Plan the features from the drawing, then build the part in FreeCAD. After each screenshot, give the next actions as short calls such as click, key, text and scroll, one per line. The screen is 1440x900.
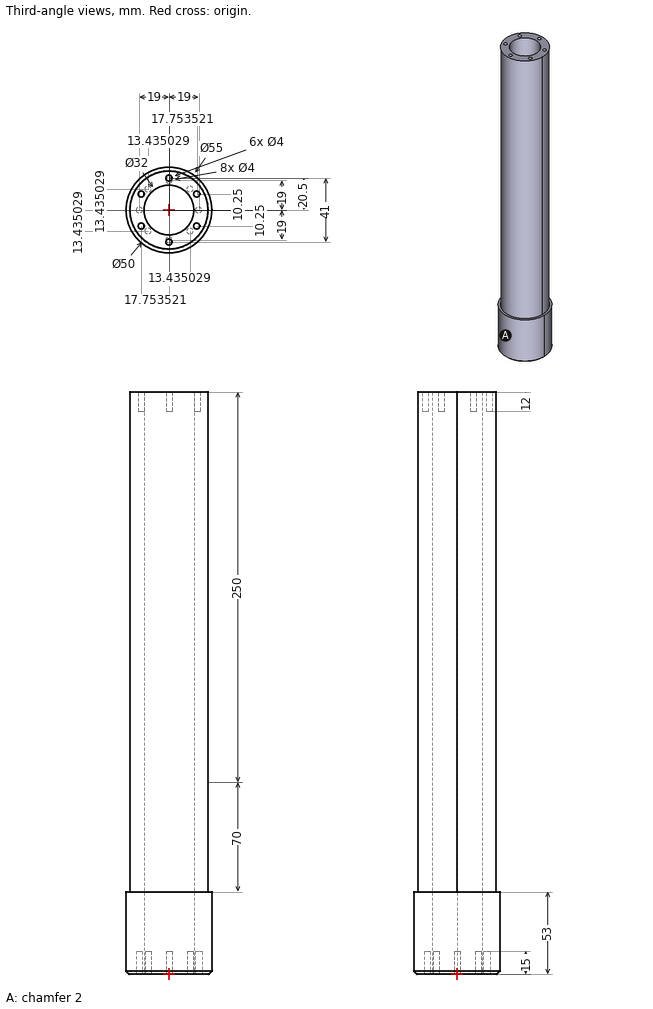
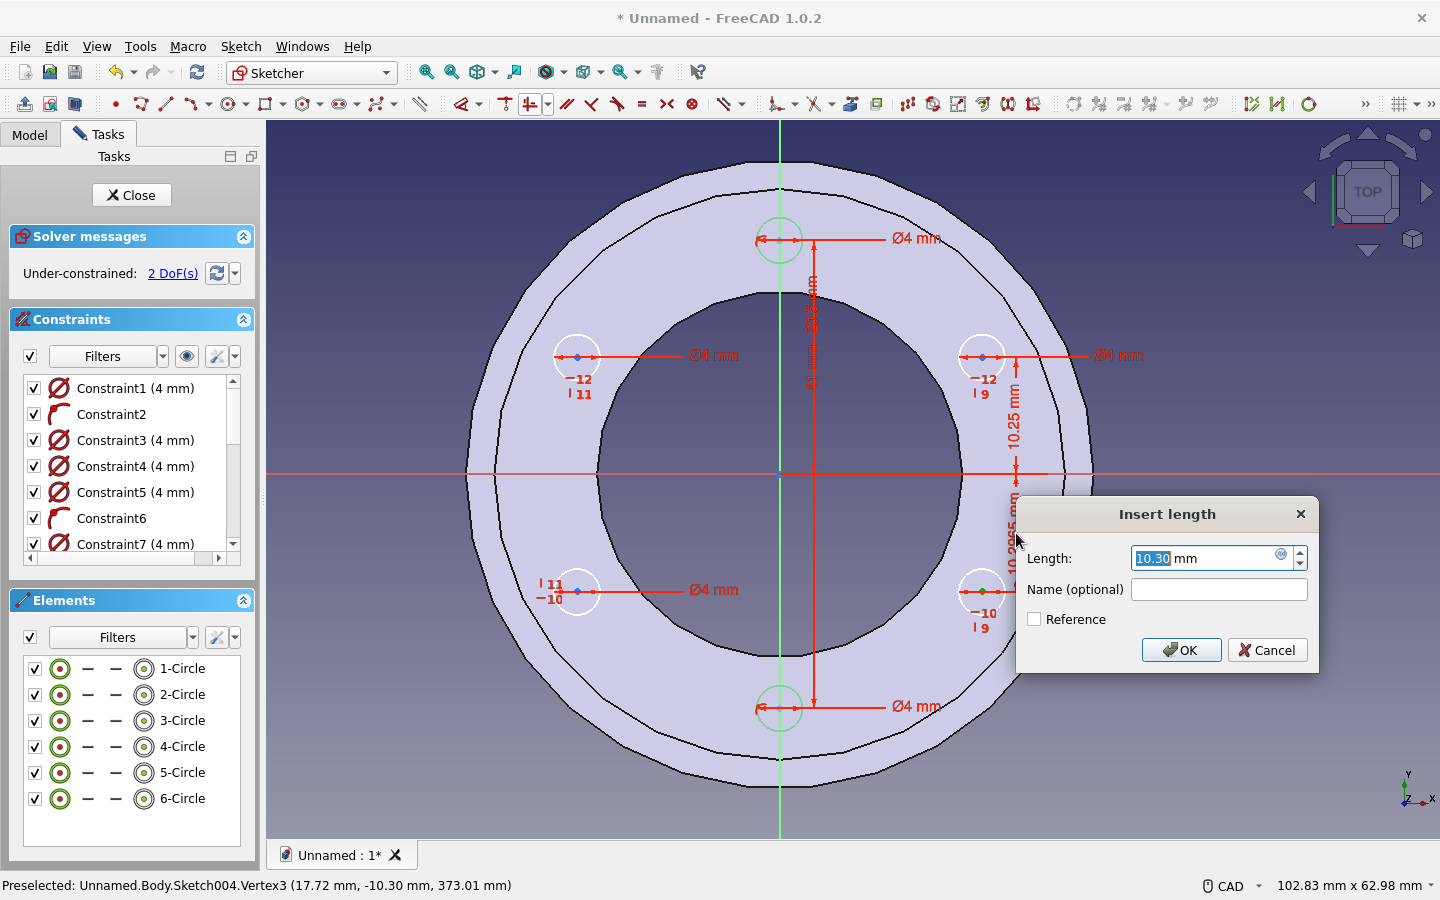
text(10.25)
key(Return)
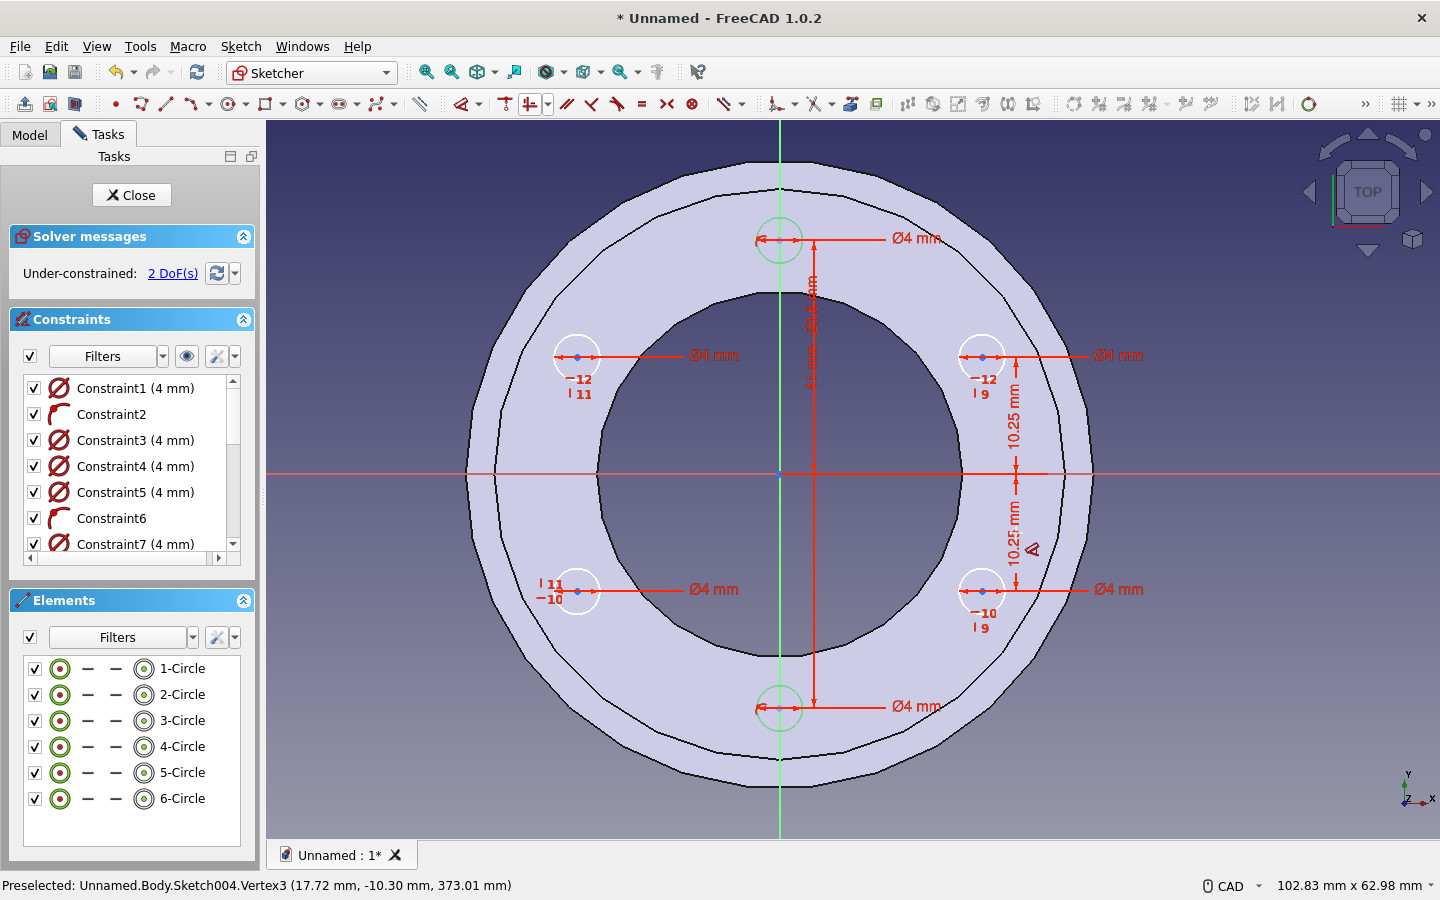
click(982, 357)
click(927, 323)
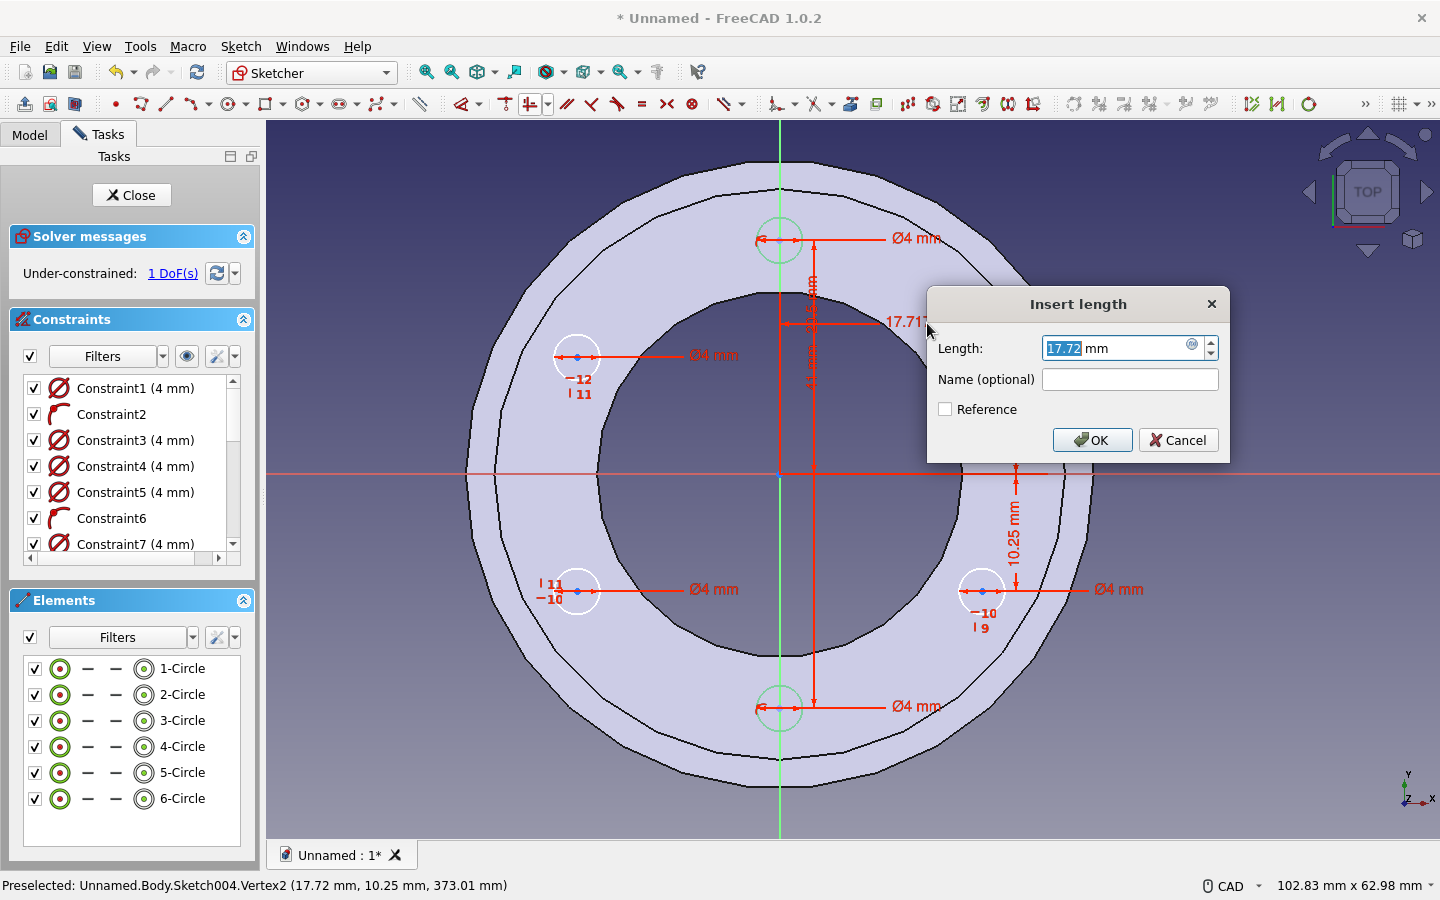
text(17.753521)
key(Return)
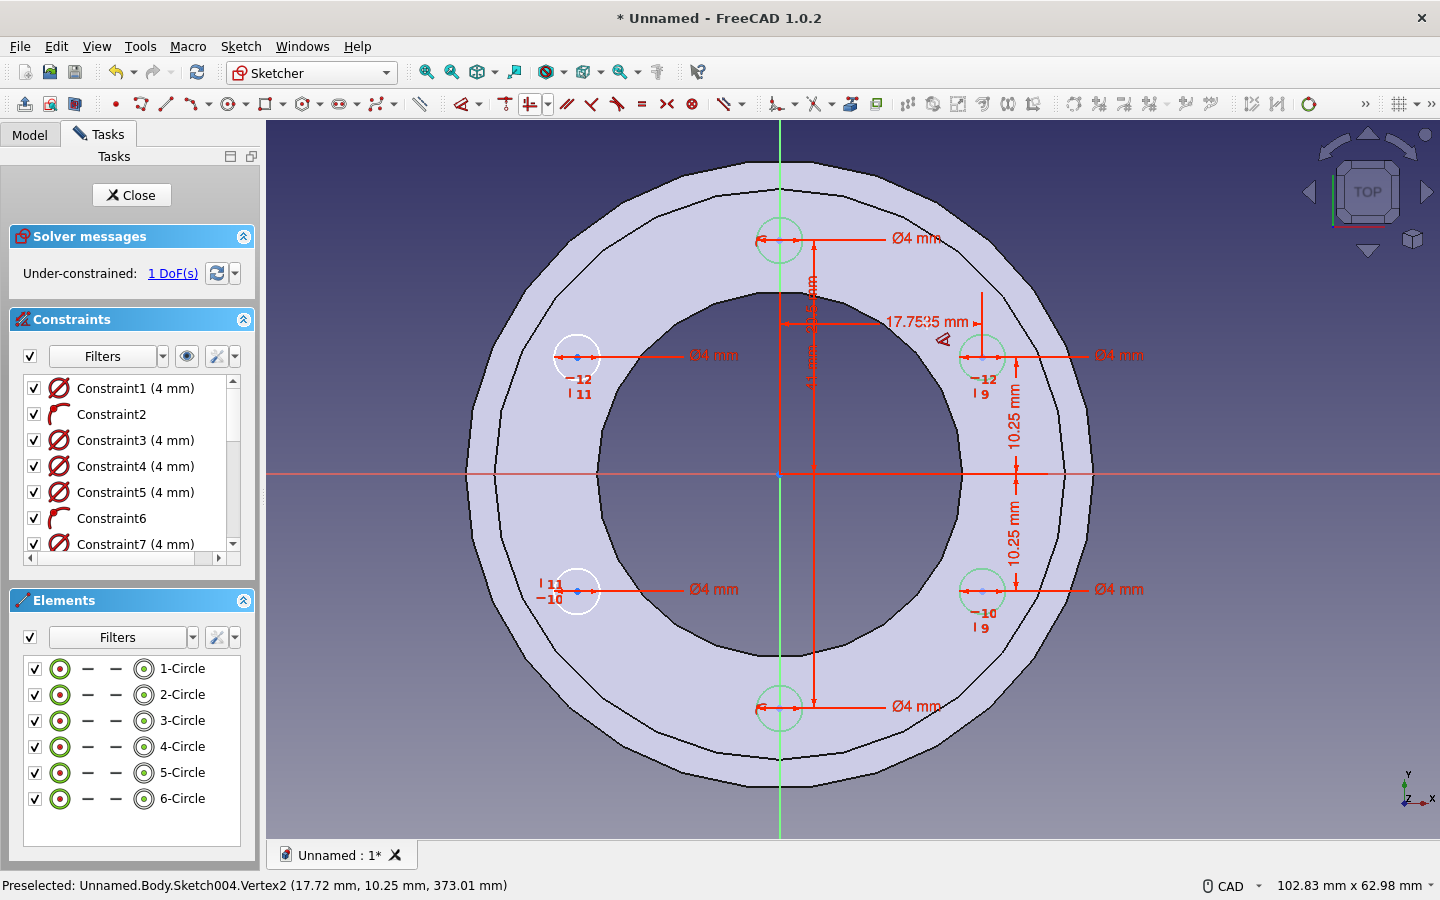
click(577, 591)
click(678, 625)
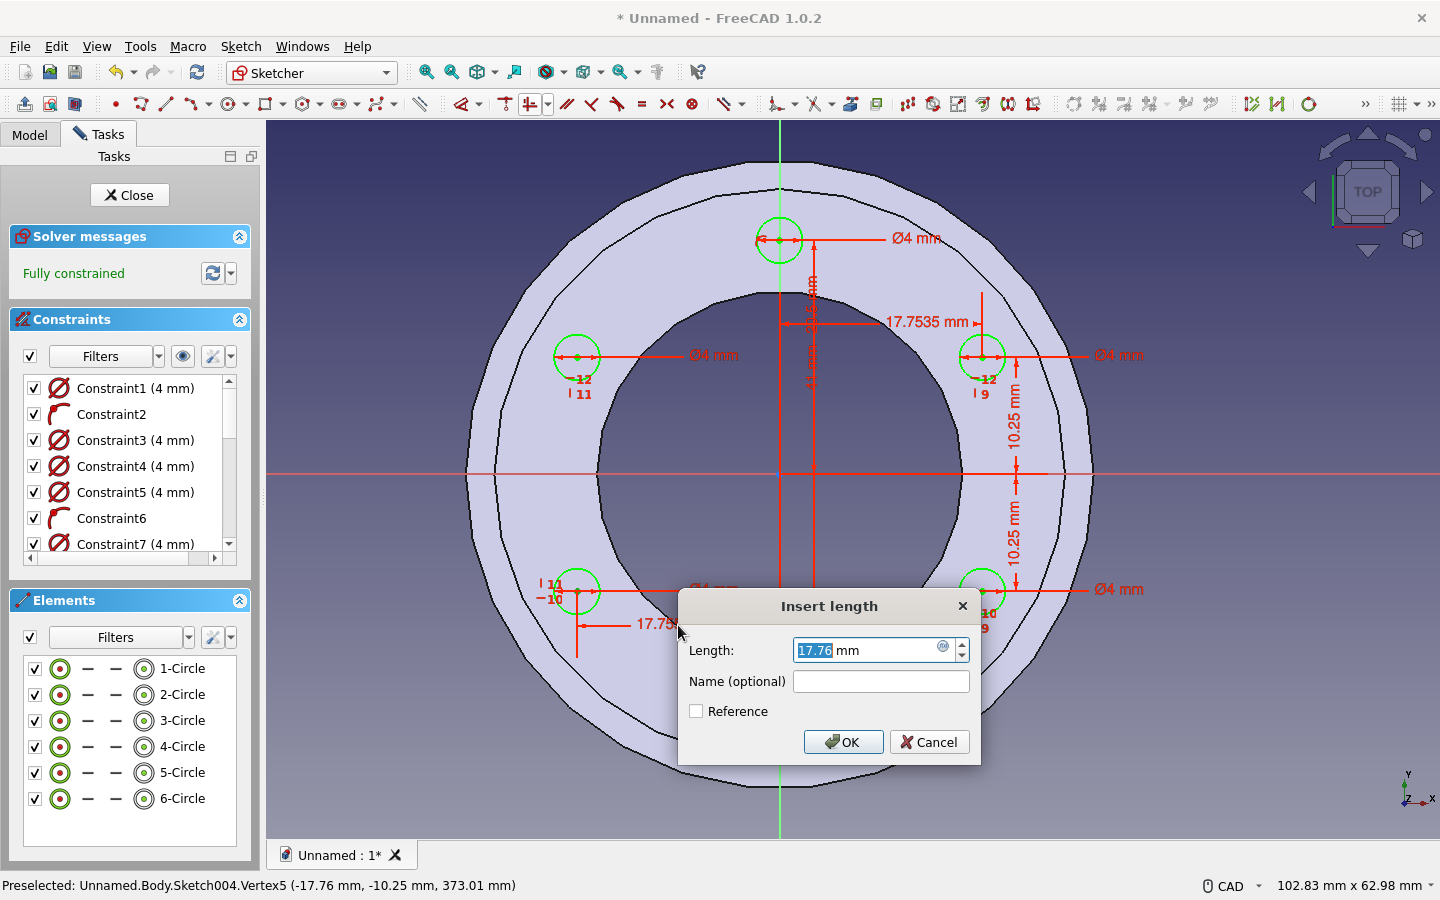
text(17.753521)
key(Return)
key(Escape)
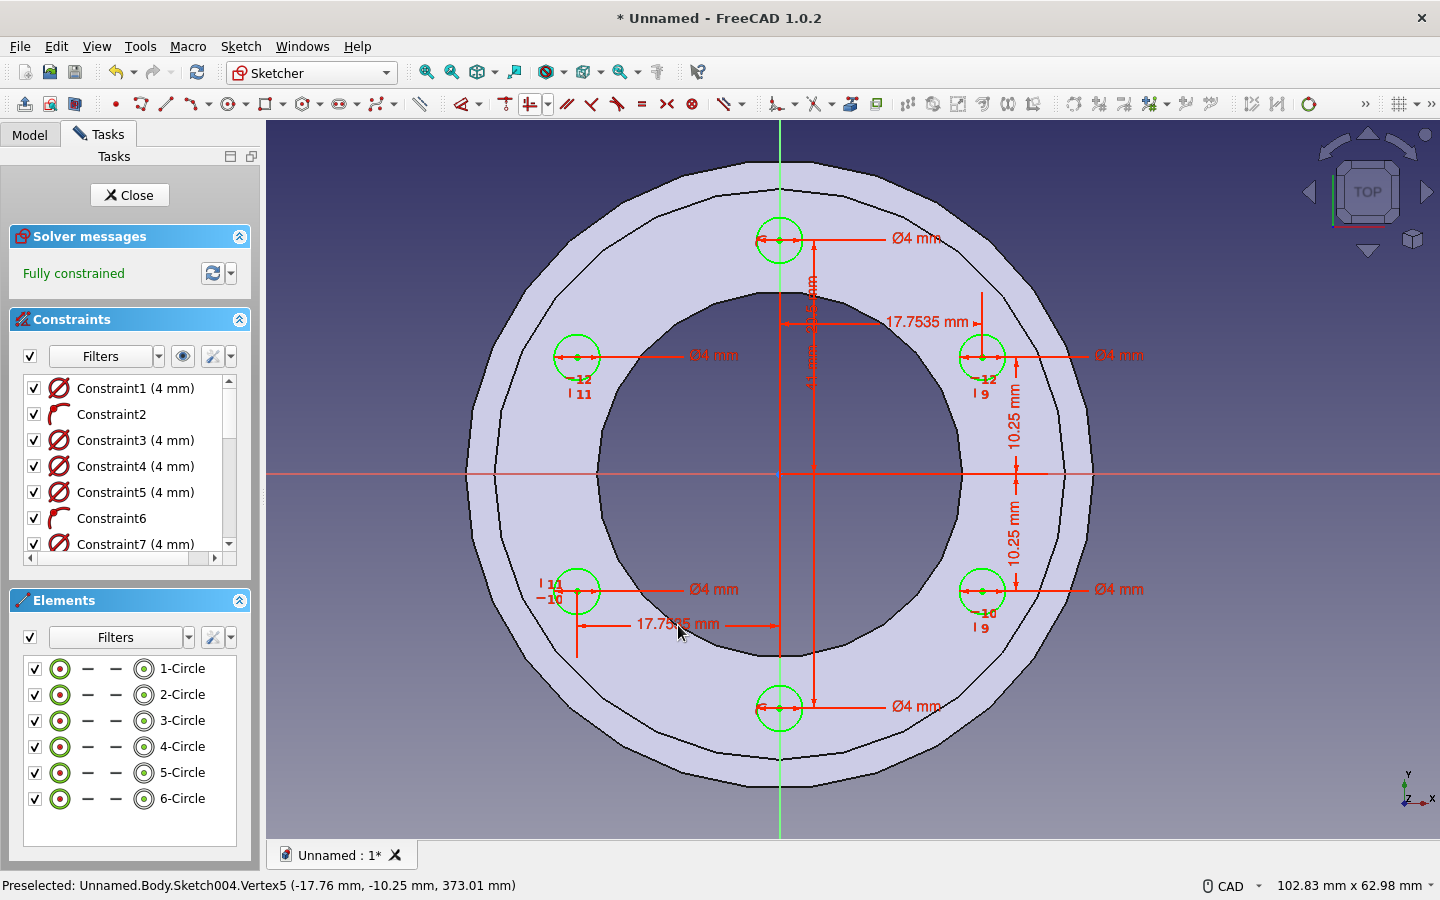
click(130, 195)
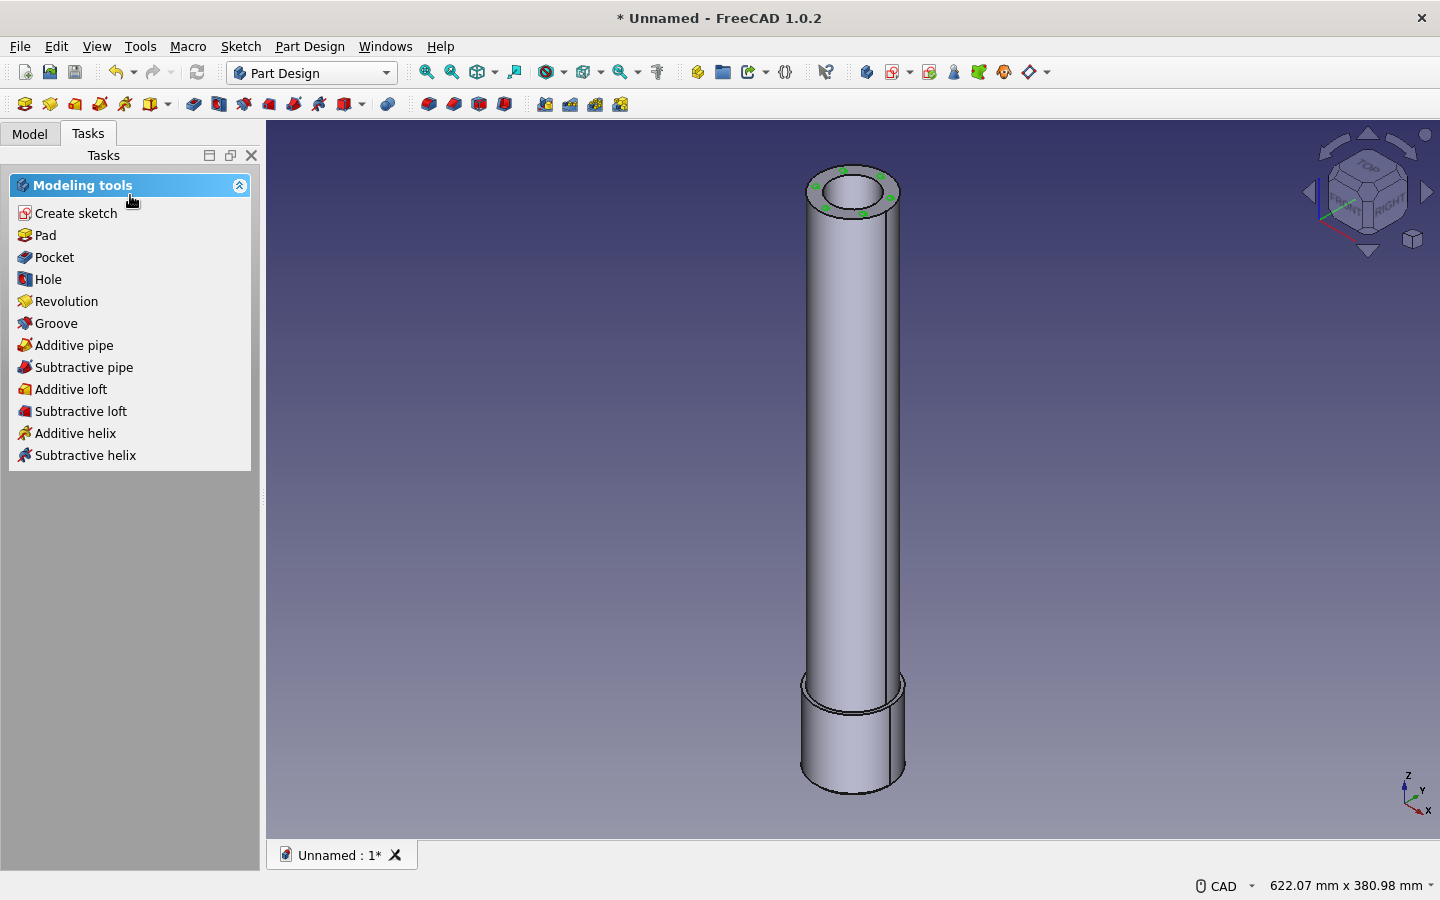
click(194, 104)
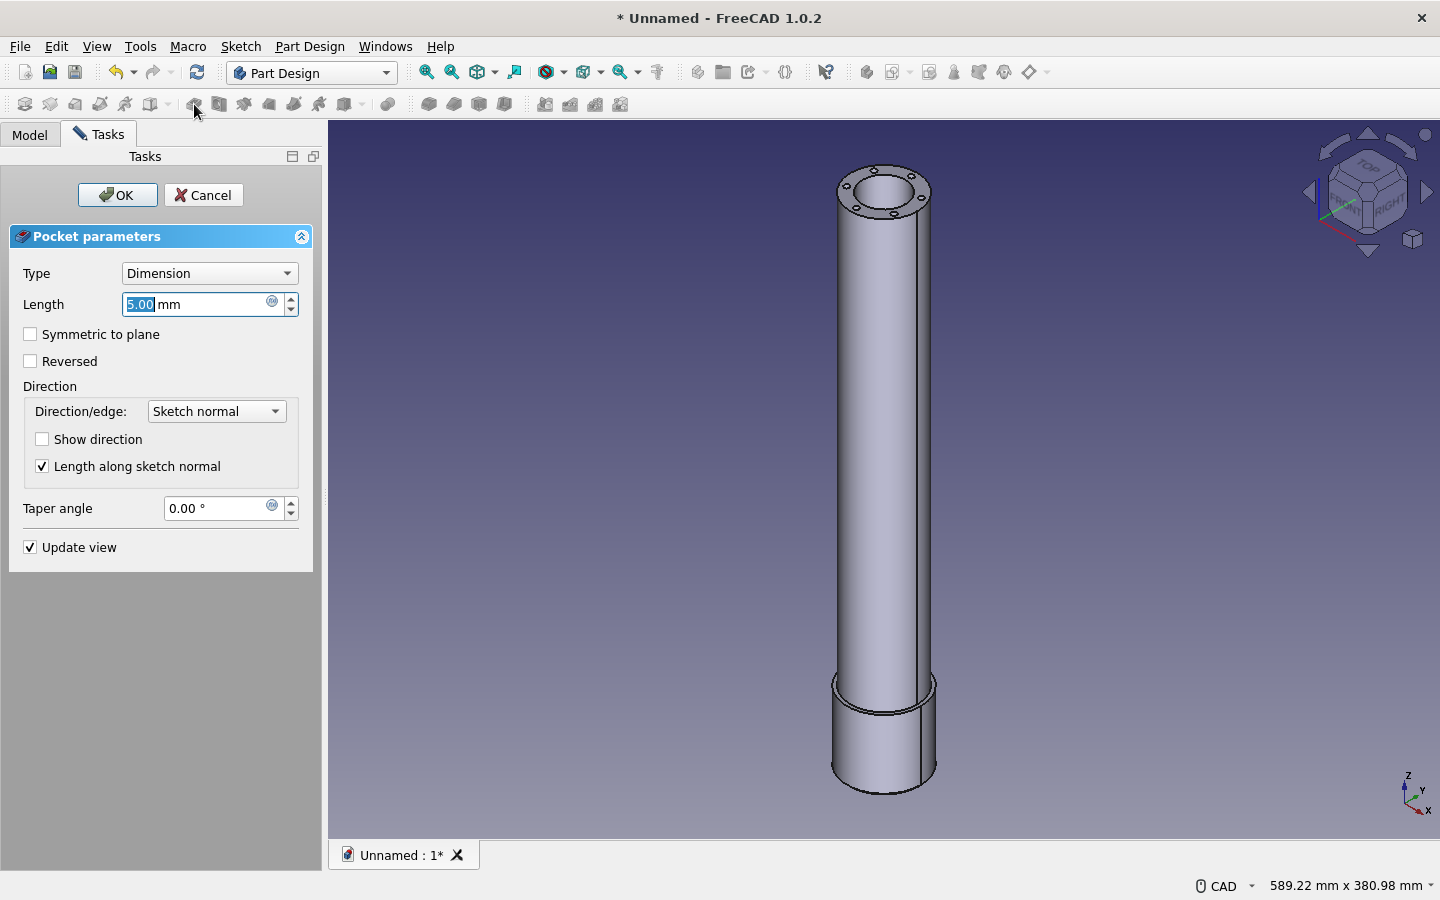
text(12)
key(Tab)